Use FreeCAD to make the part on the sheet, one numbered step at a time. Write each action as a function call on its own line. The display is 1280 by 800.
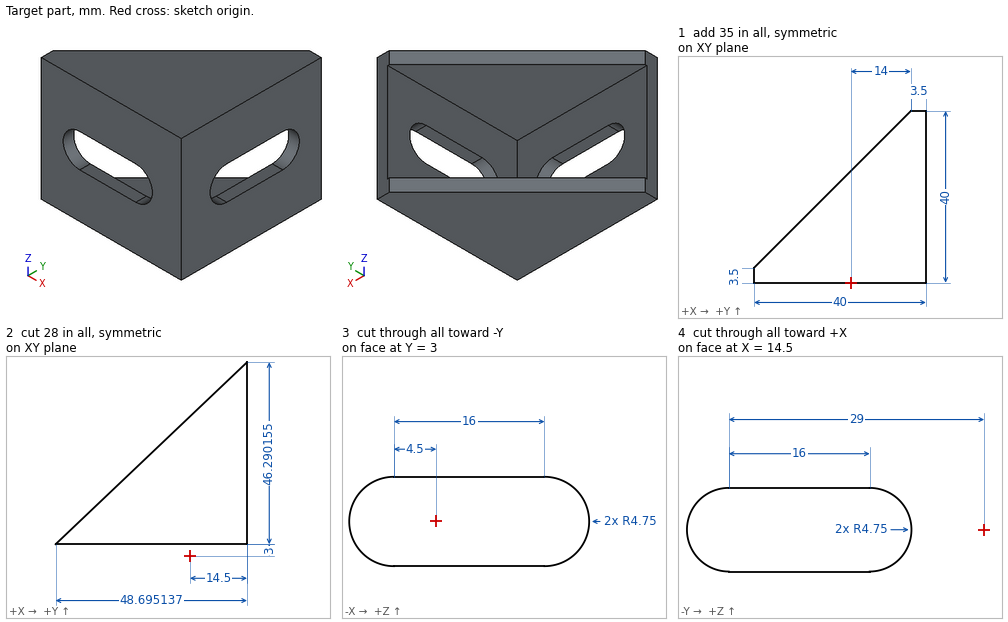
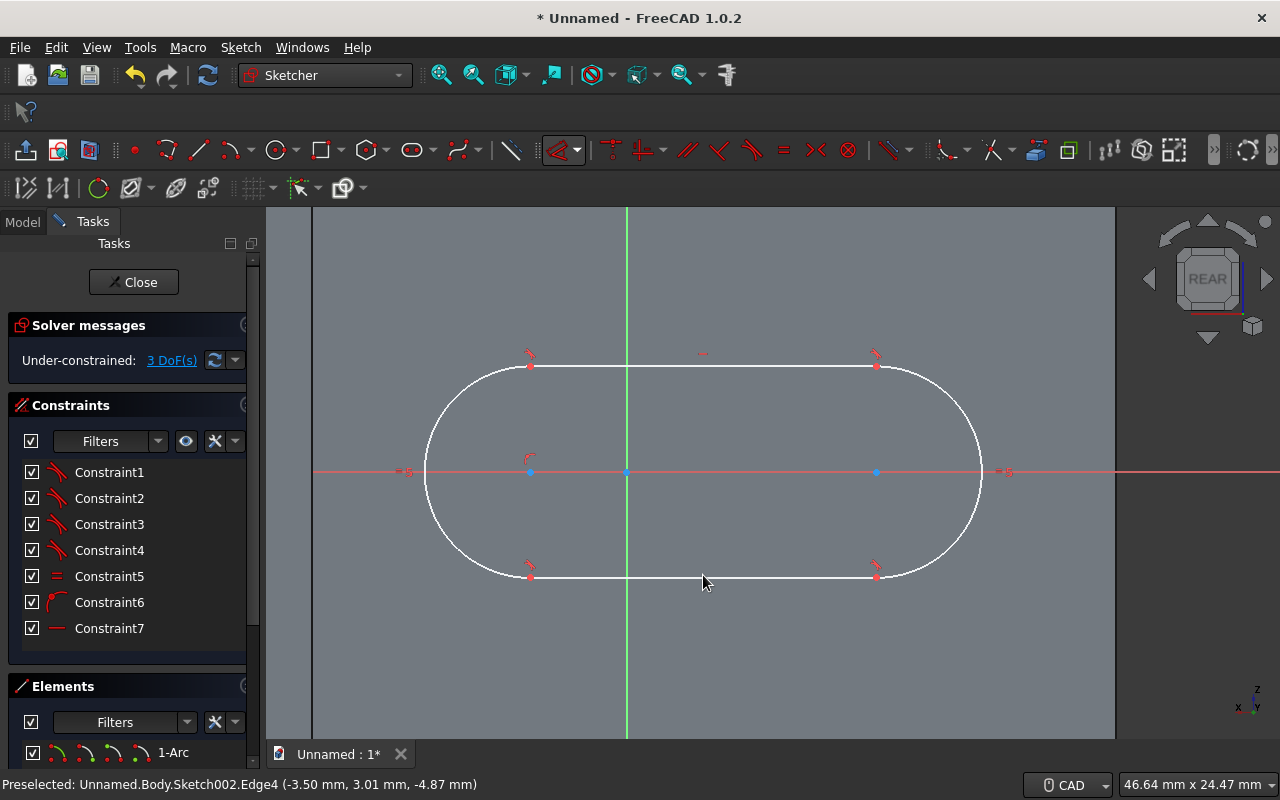
click(445, 410)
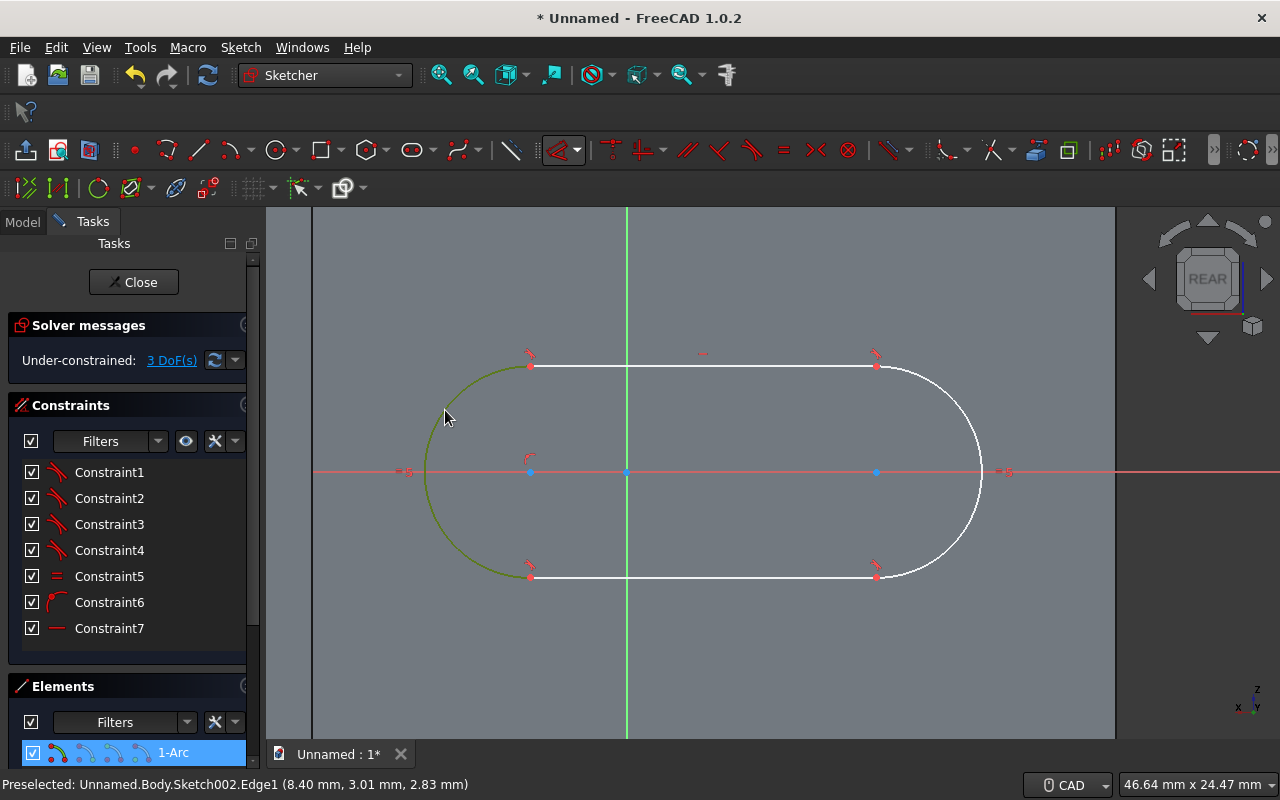
key(k)
key(r)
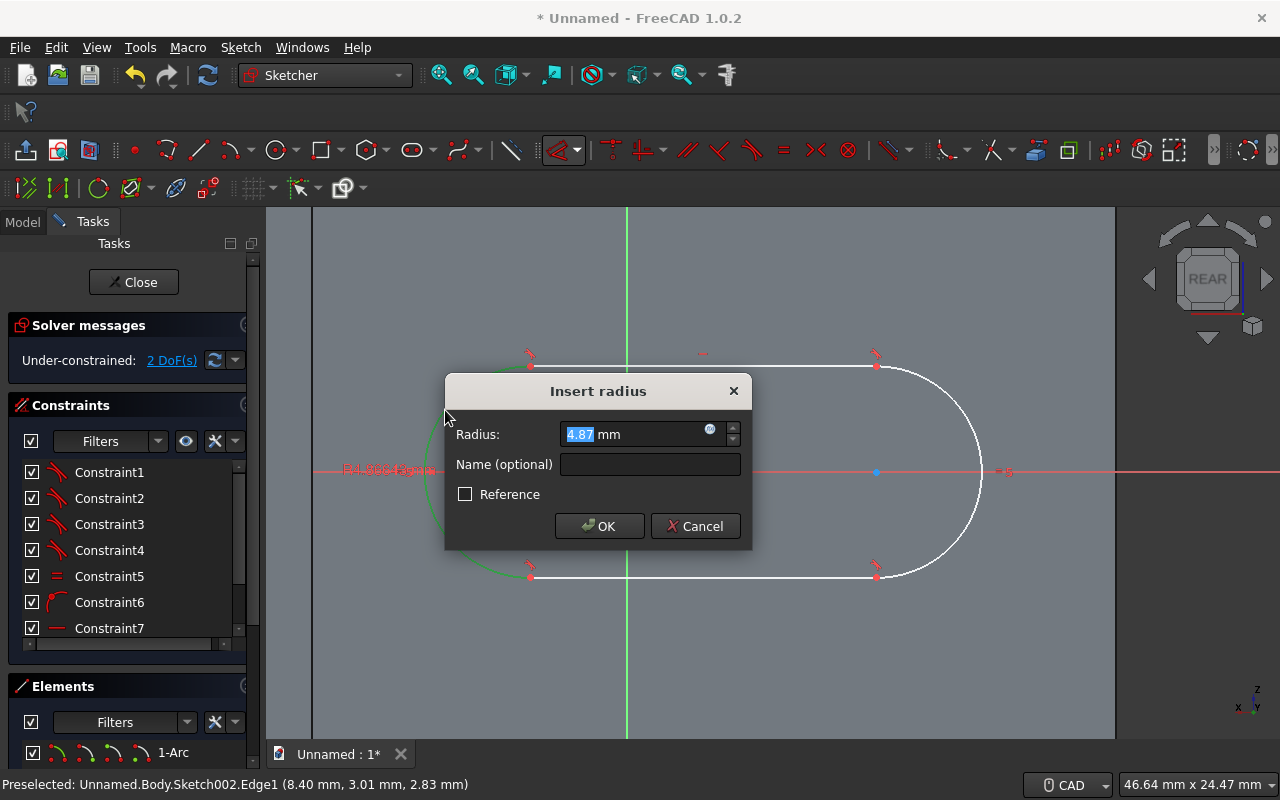
text(4.75)
key(Return)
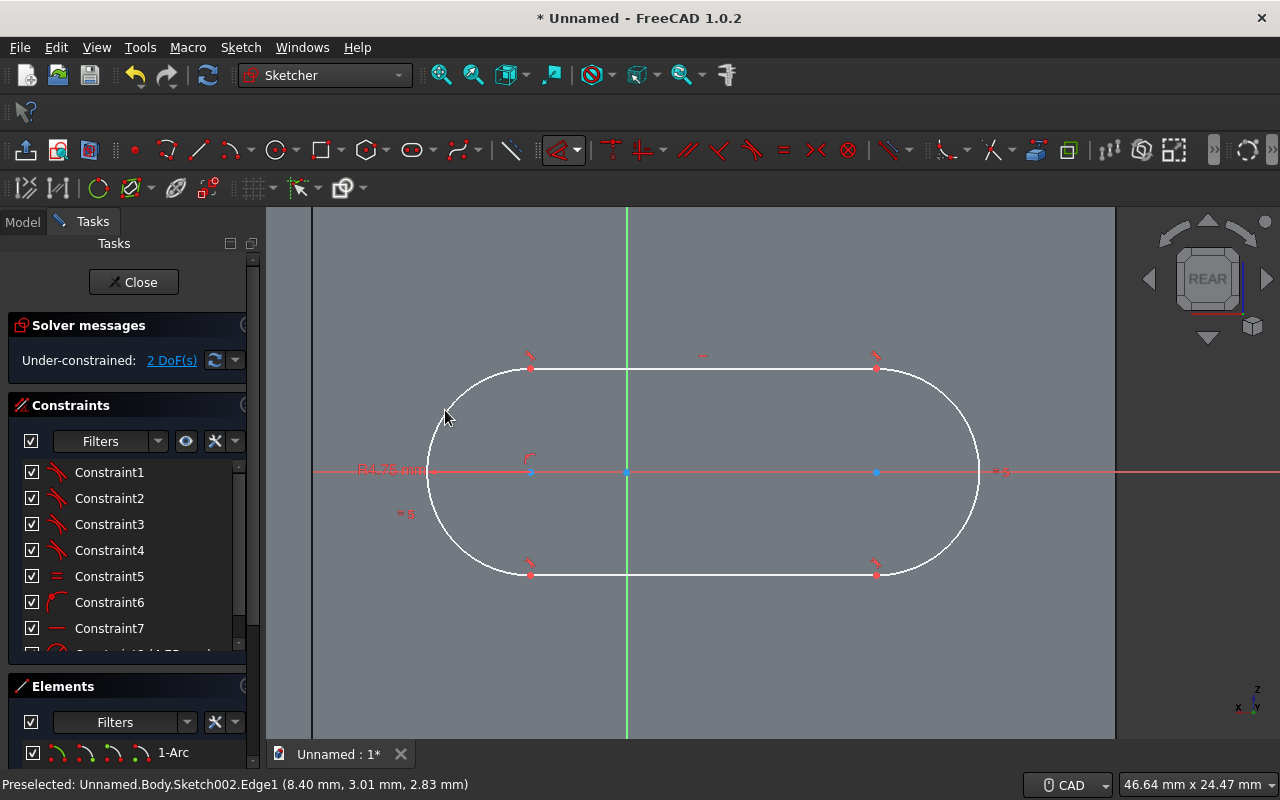
click(772, 369)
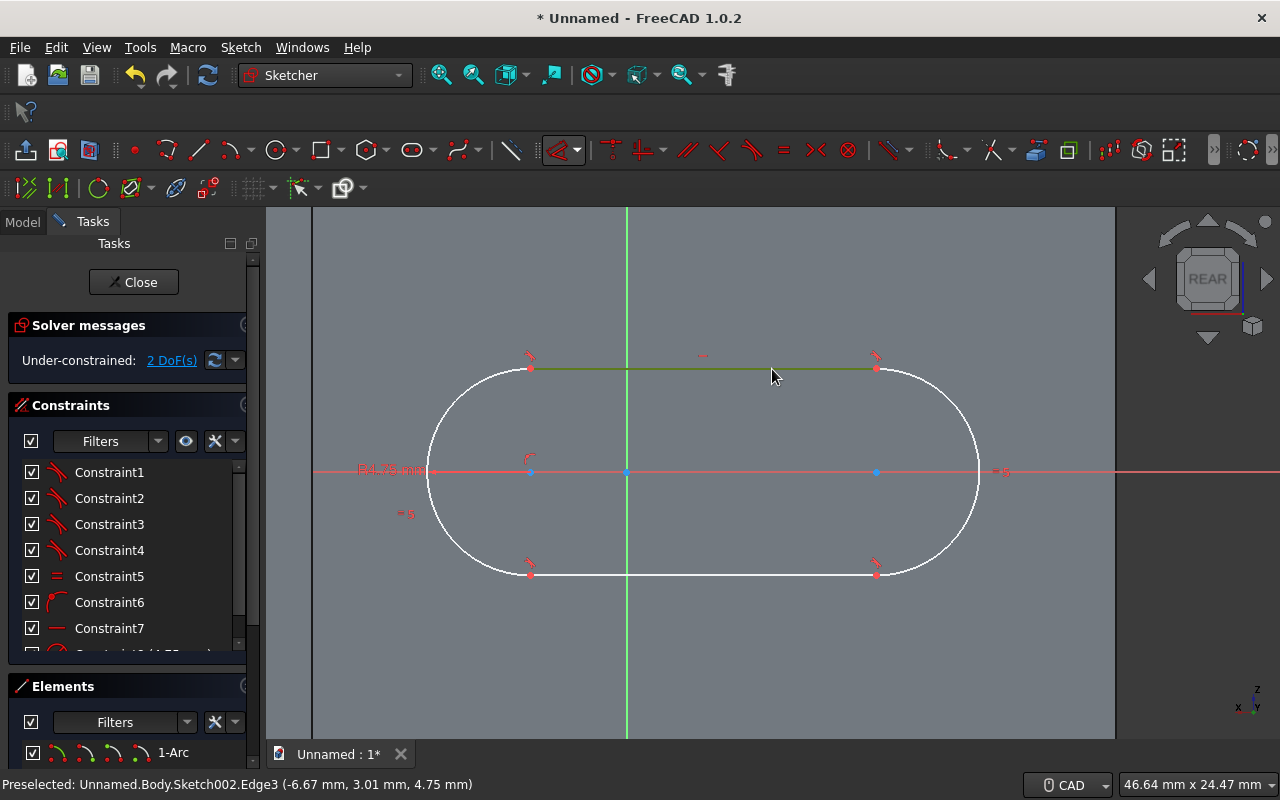
key(l)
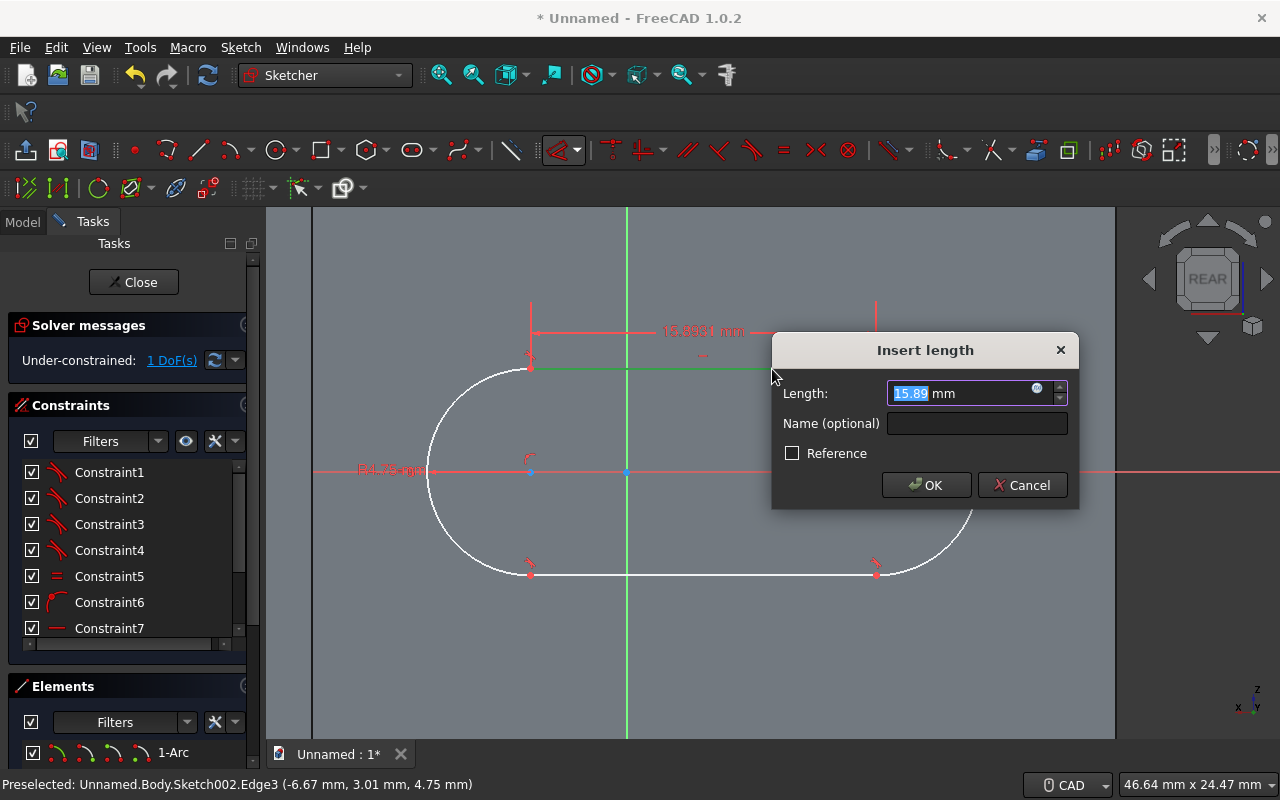
text(16)
key(Return)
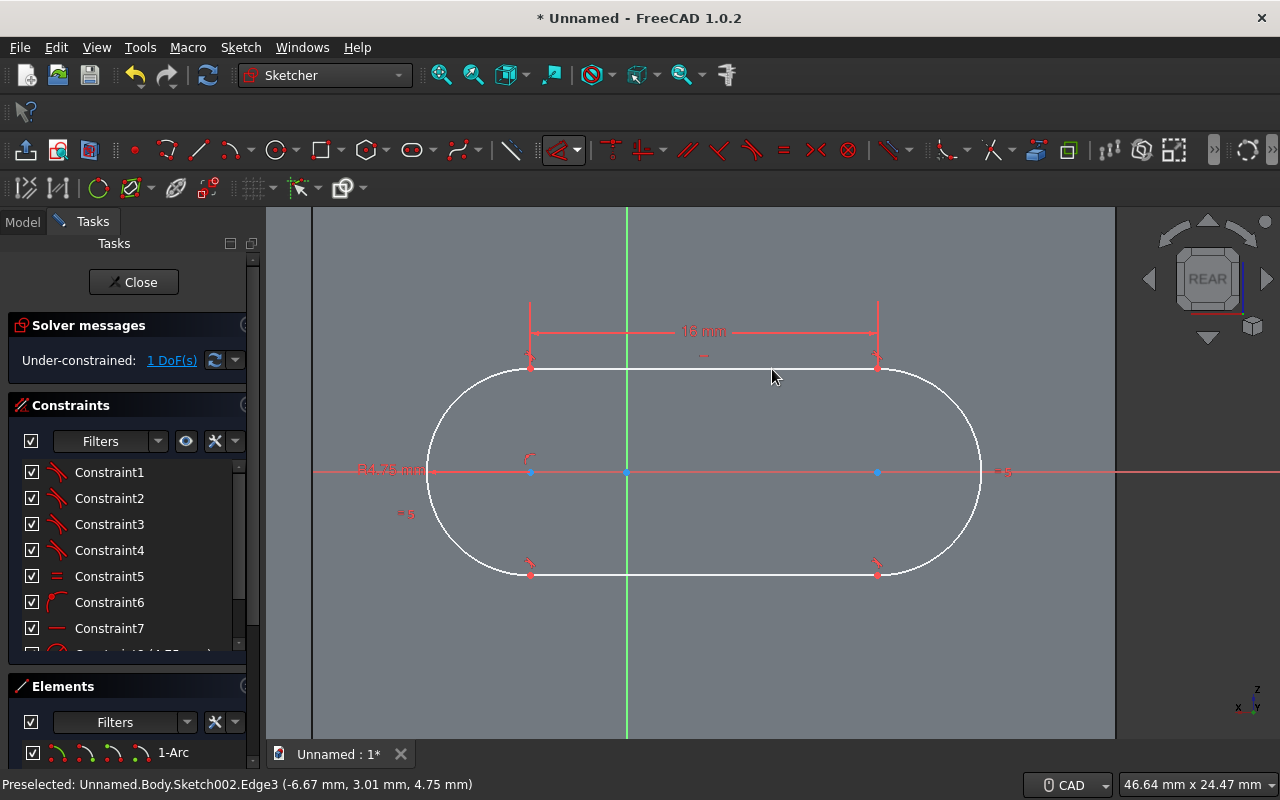
click(530, 369)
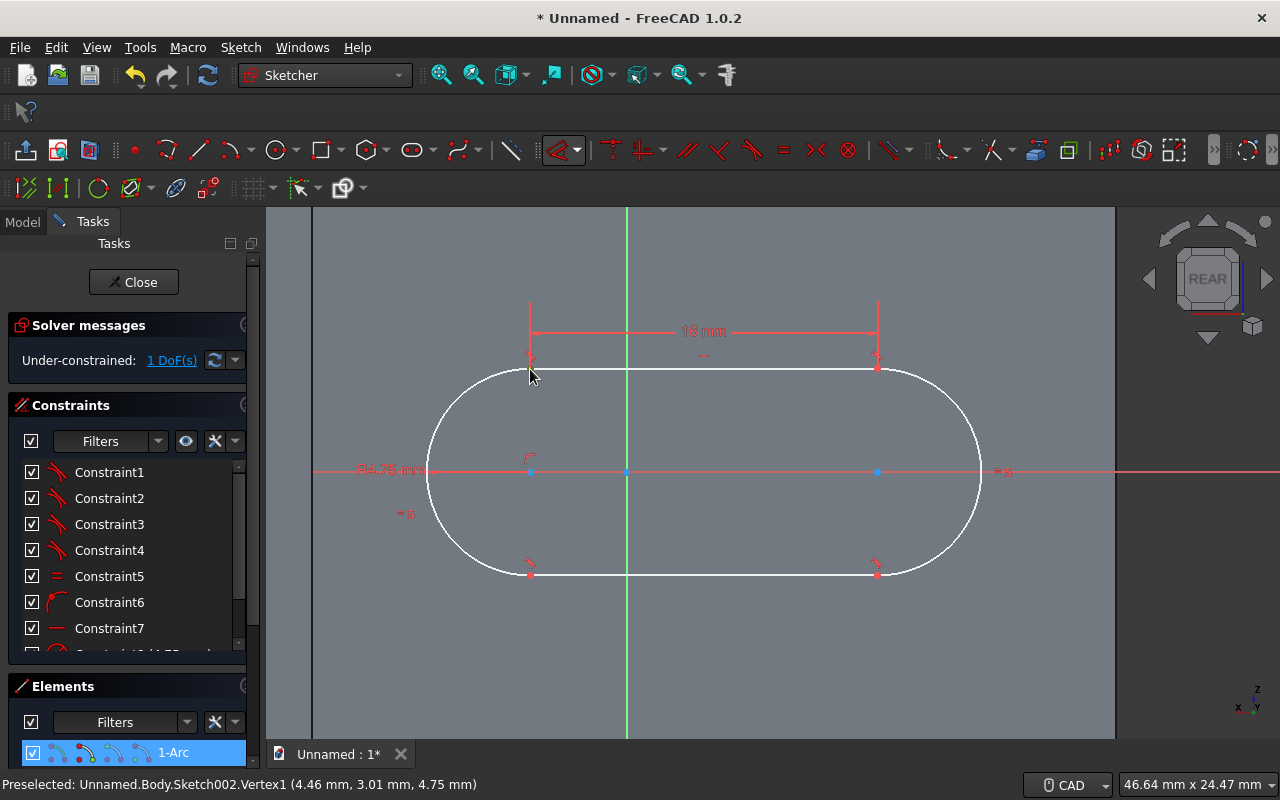
click(580, 150)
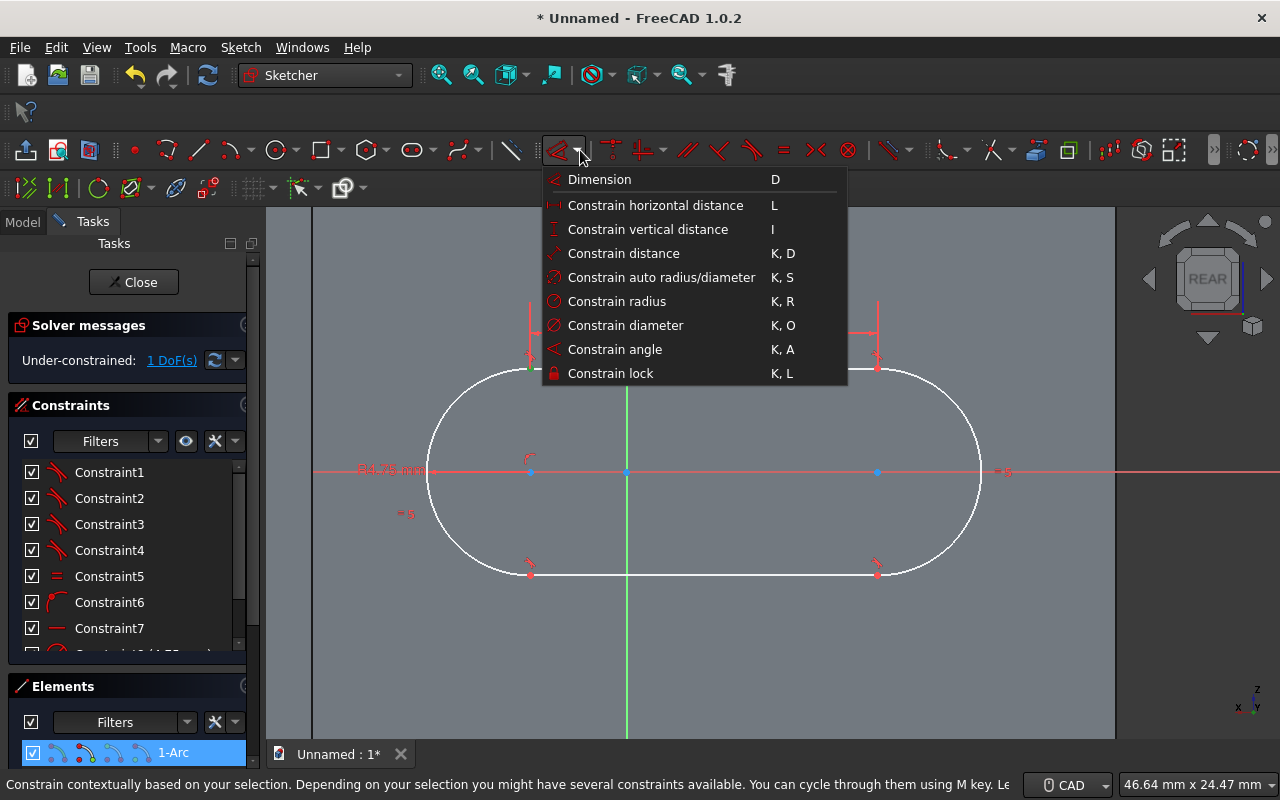
click(695, 205)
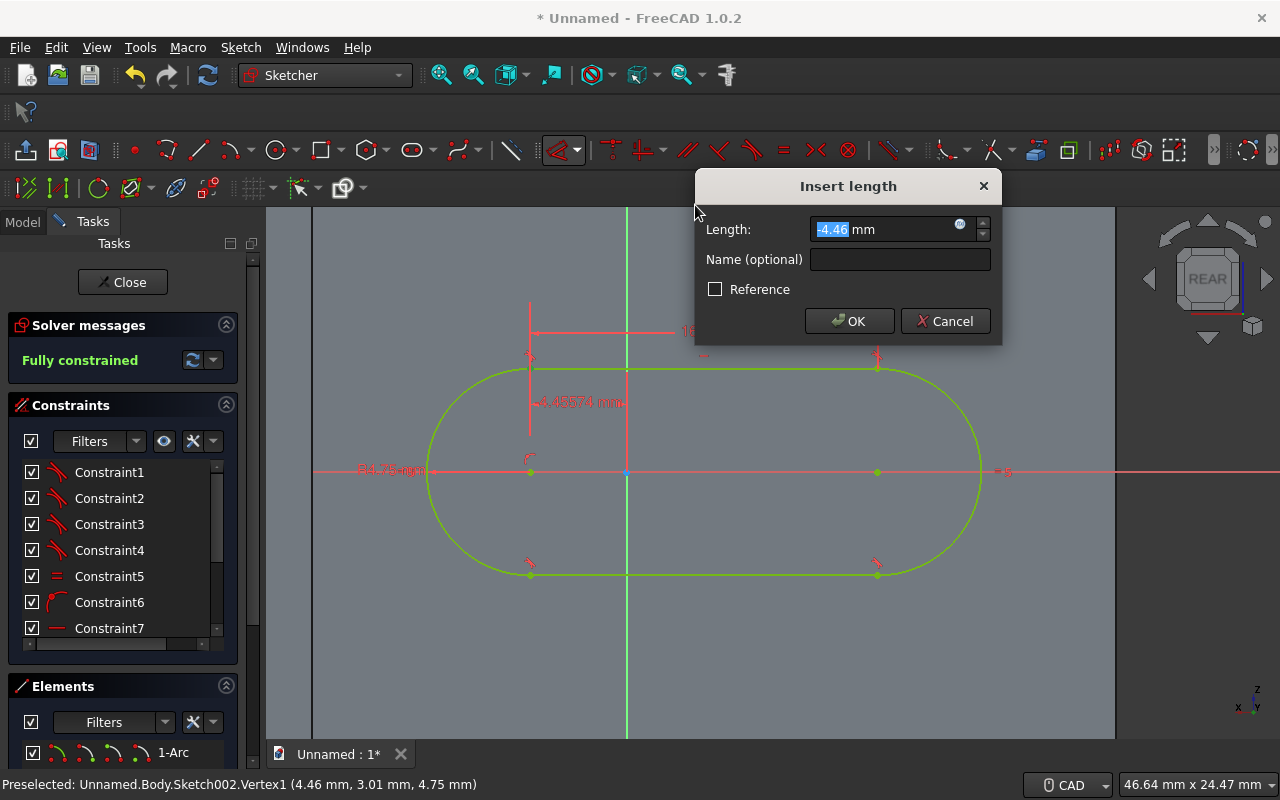
text(-4.5)
key(Return)